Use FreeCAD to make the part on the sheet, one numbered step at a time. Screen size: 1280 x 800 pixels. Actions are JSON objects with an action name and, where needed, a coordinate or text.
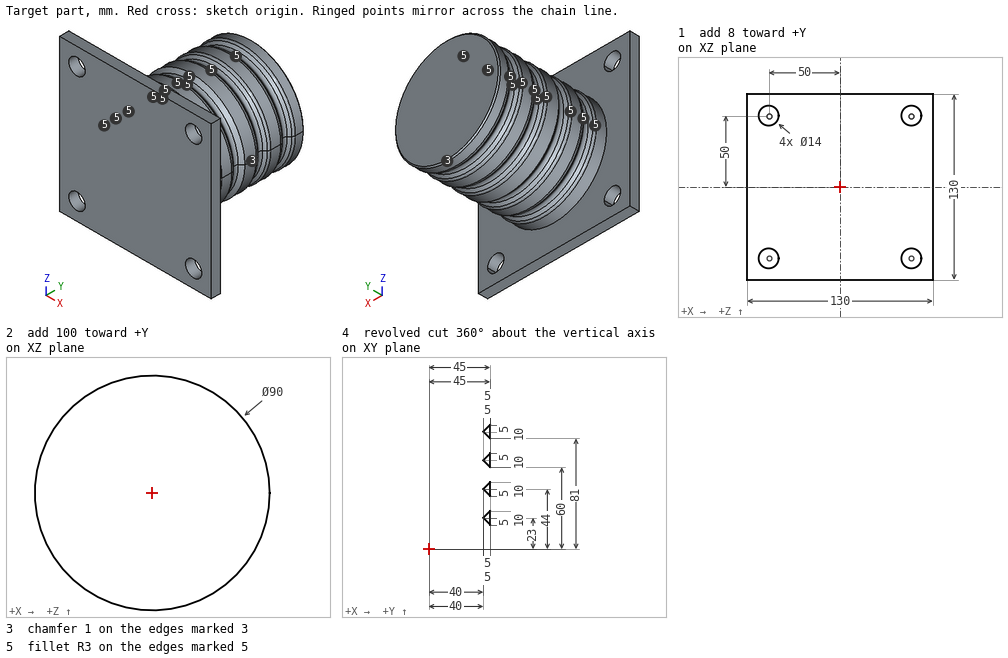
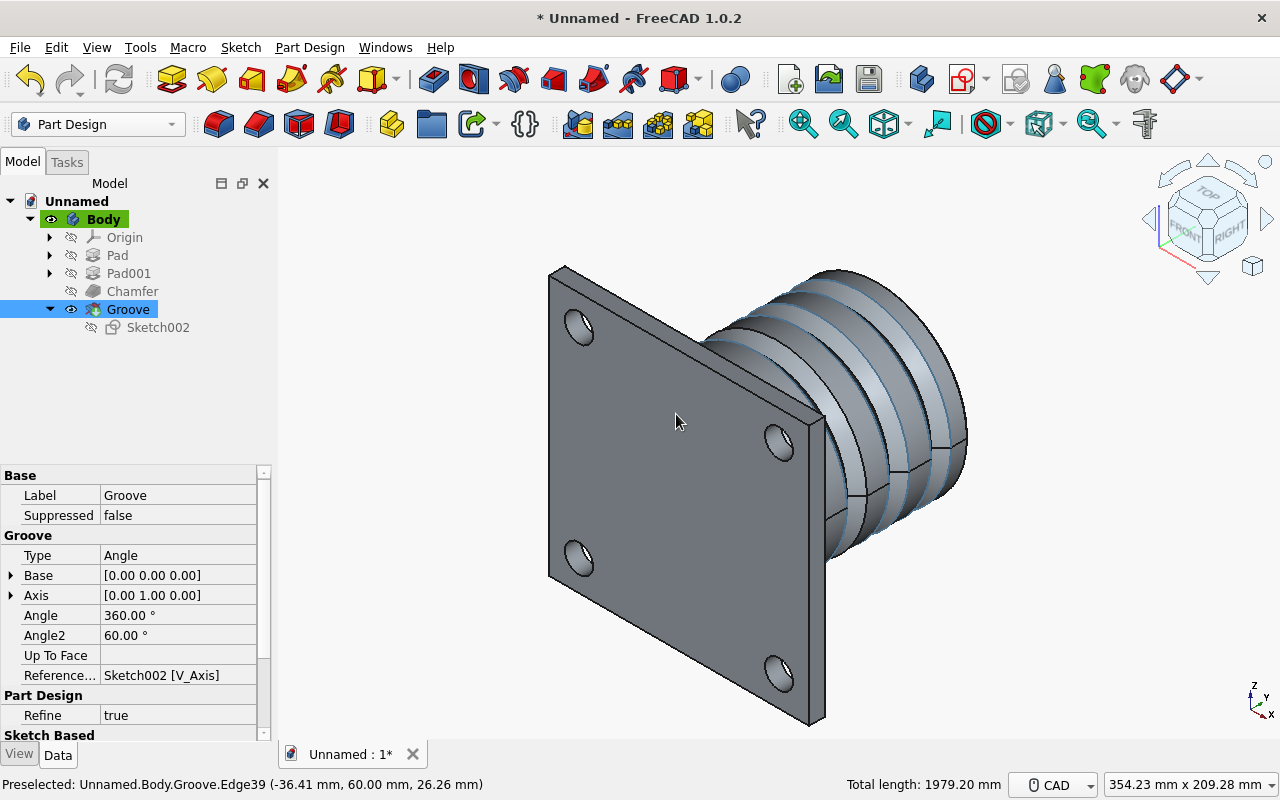
{"action": "key", "text": "1"}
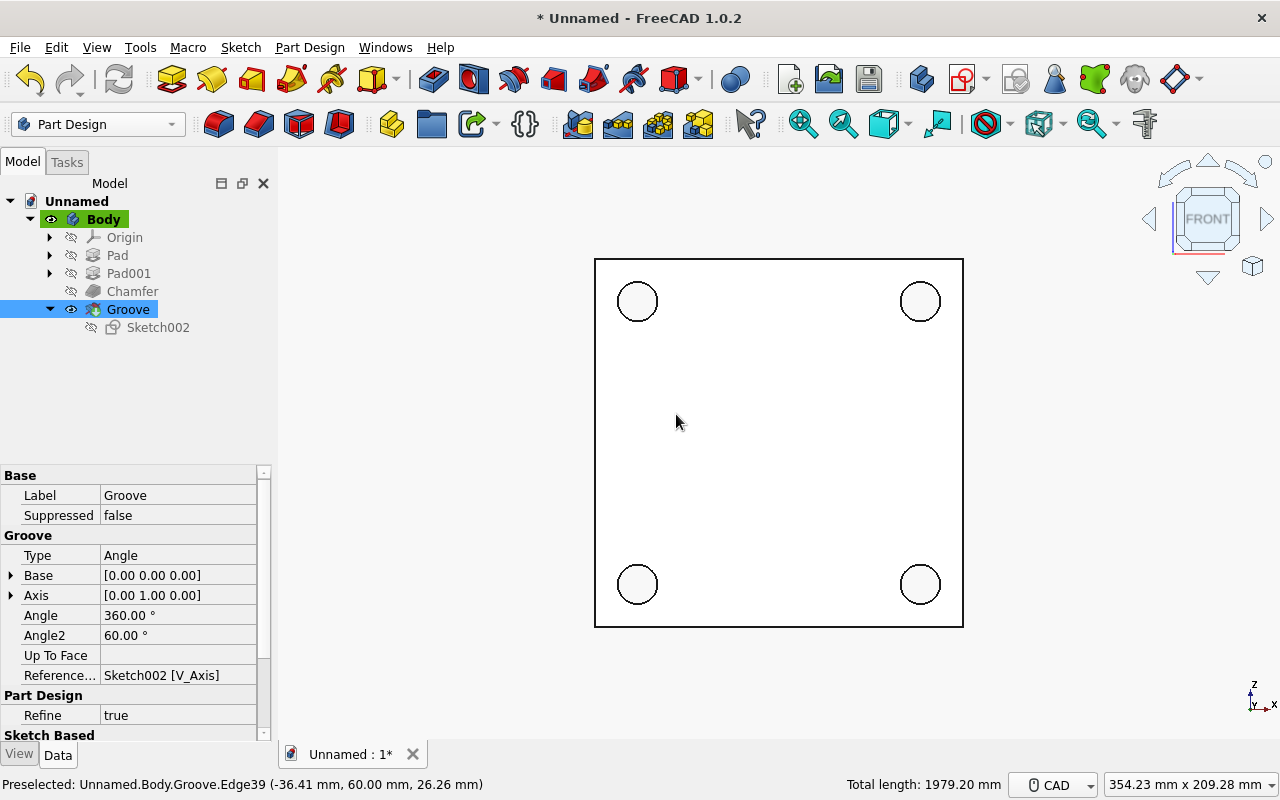
{"action": "key", "text": "3"}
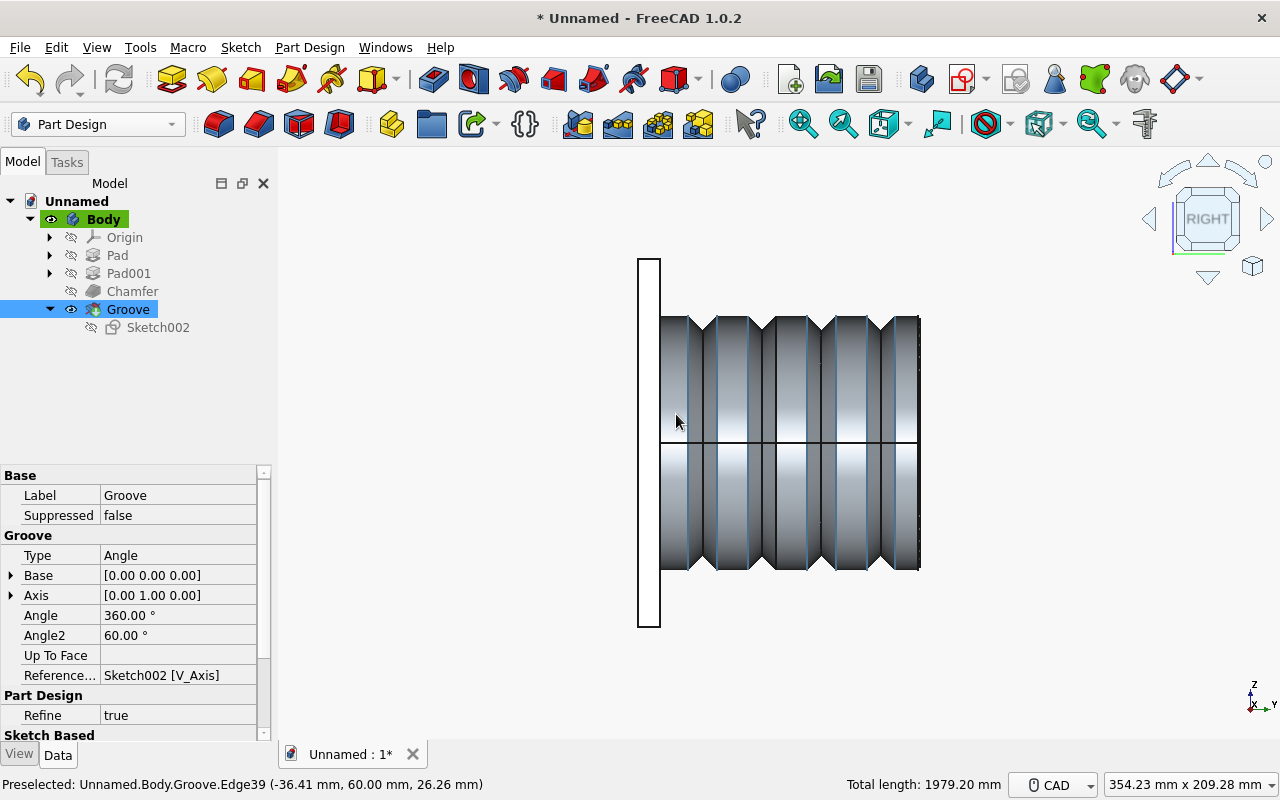
{"action": "key", "text": "5"}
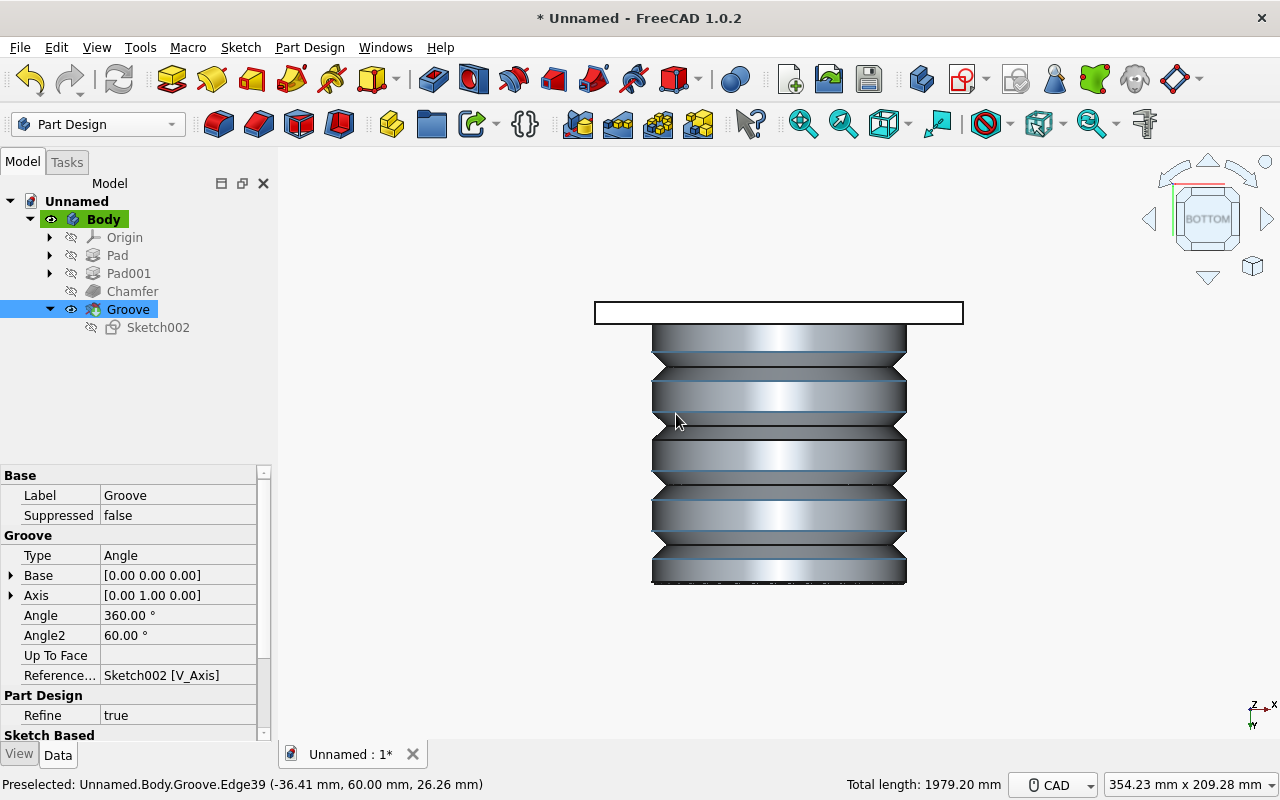
{"action": "key", "text": "4"}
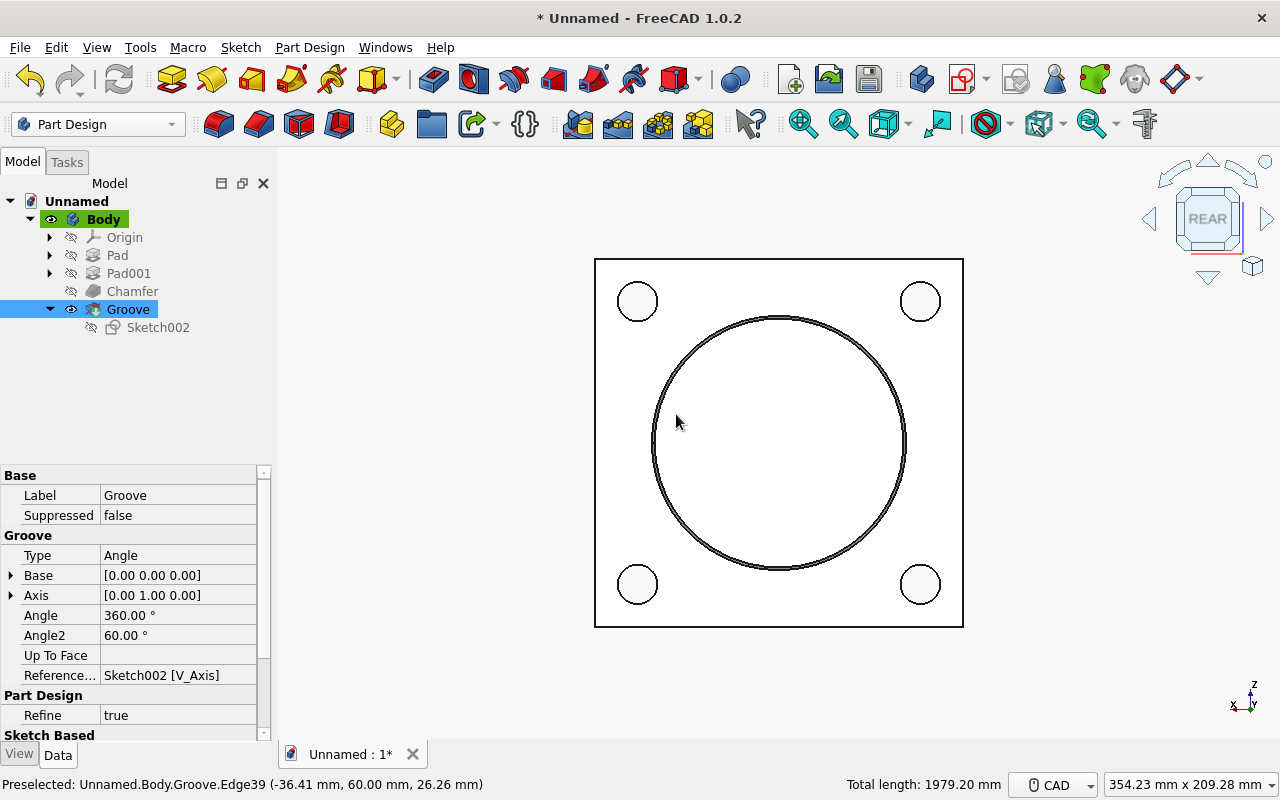
{"action": "key", "text": "6"}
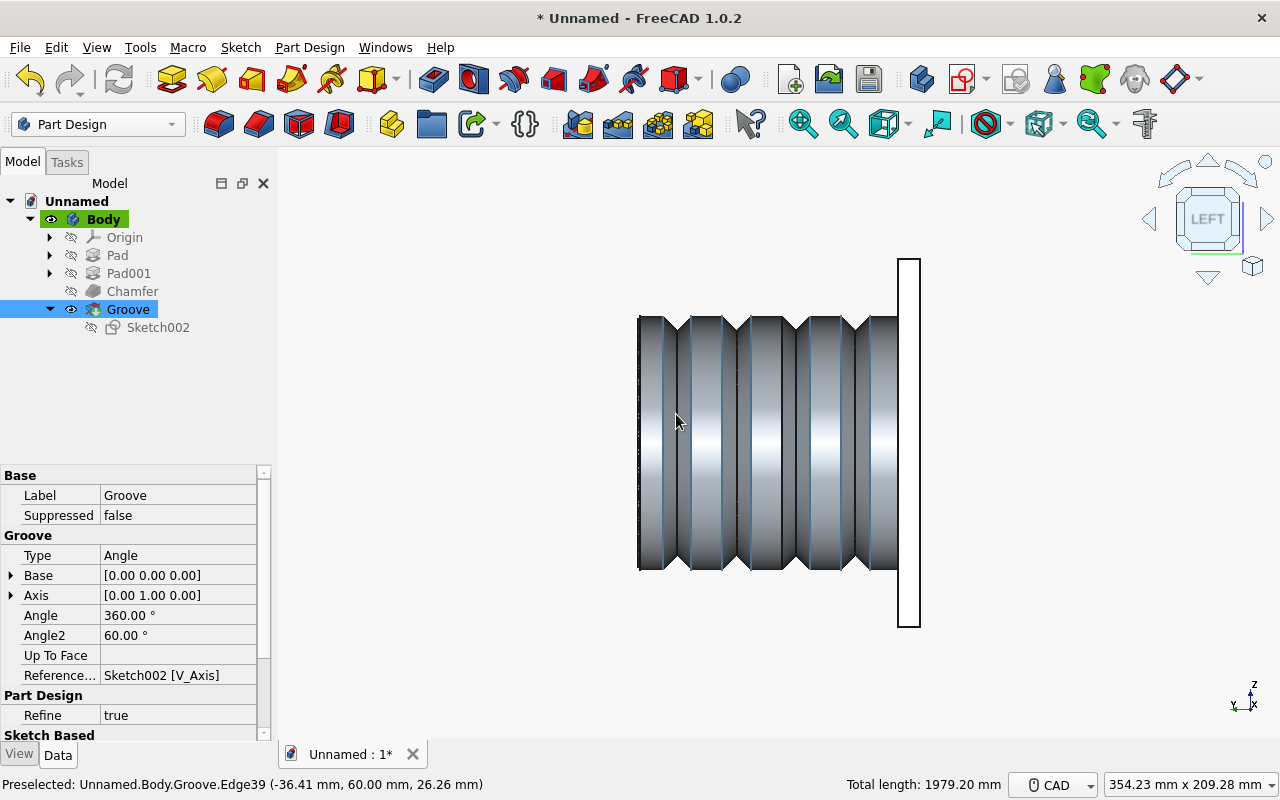
{"action": "key", "text": "v 3"}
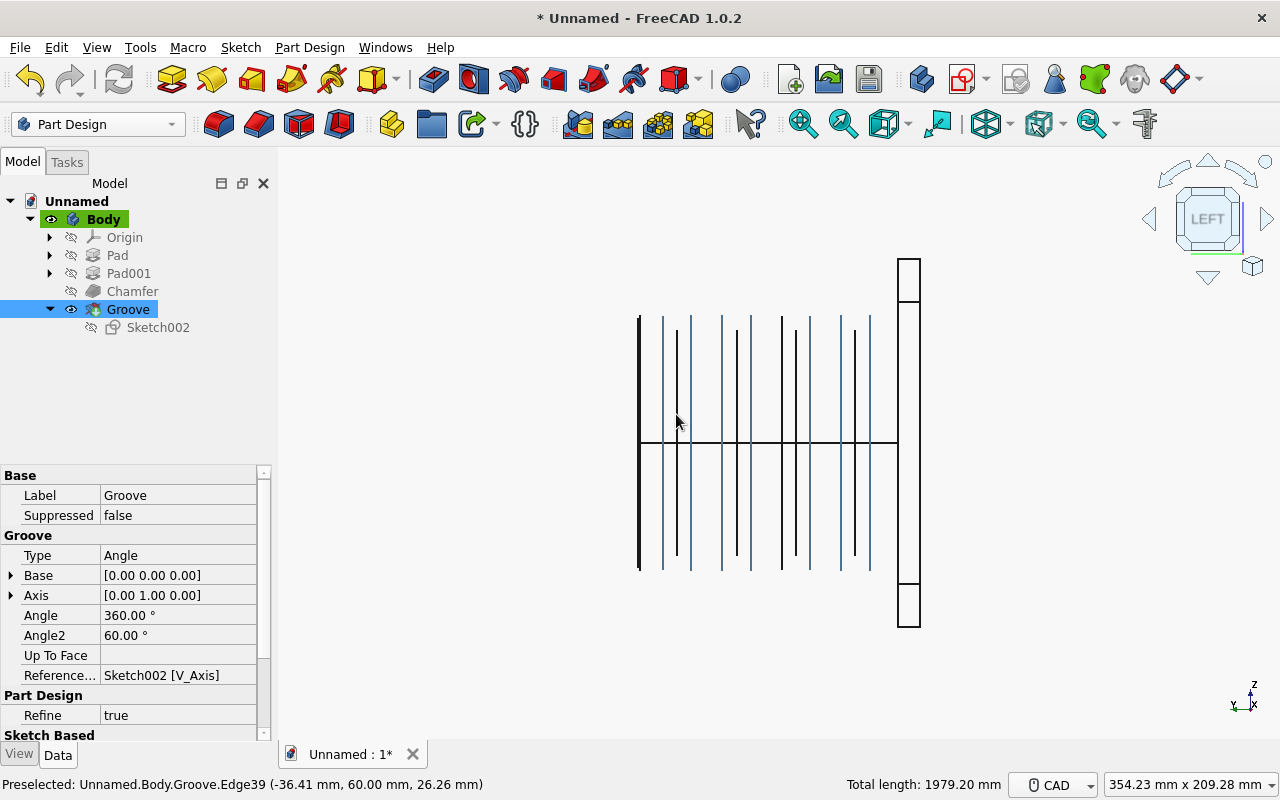
{"action": "key", "text": "0"}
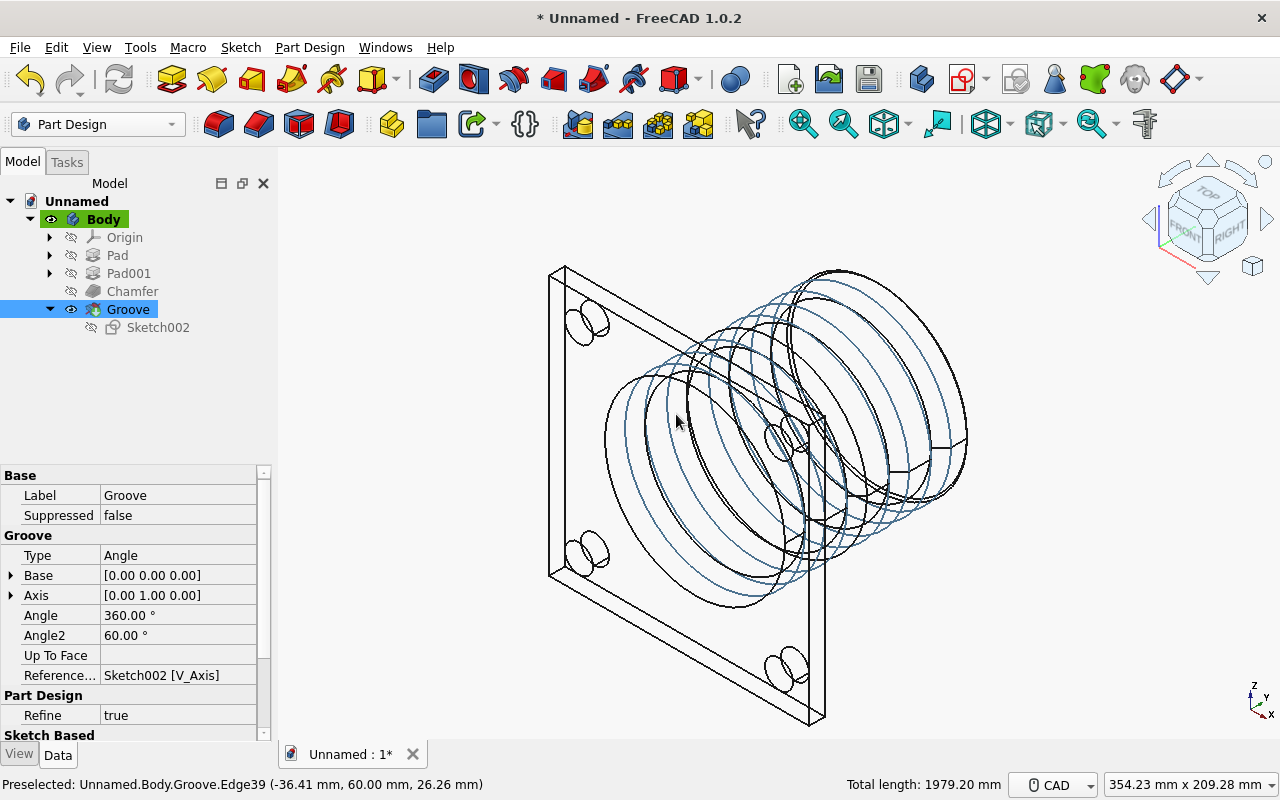
{"action": "left_click", "coordinate": [645, 427], "text": "ctrl"}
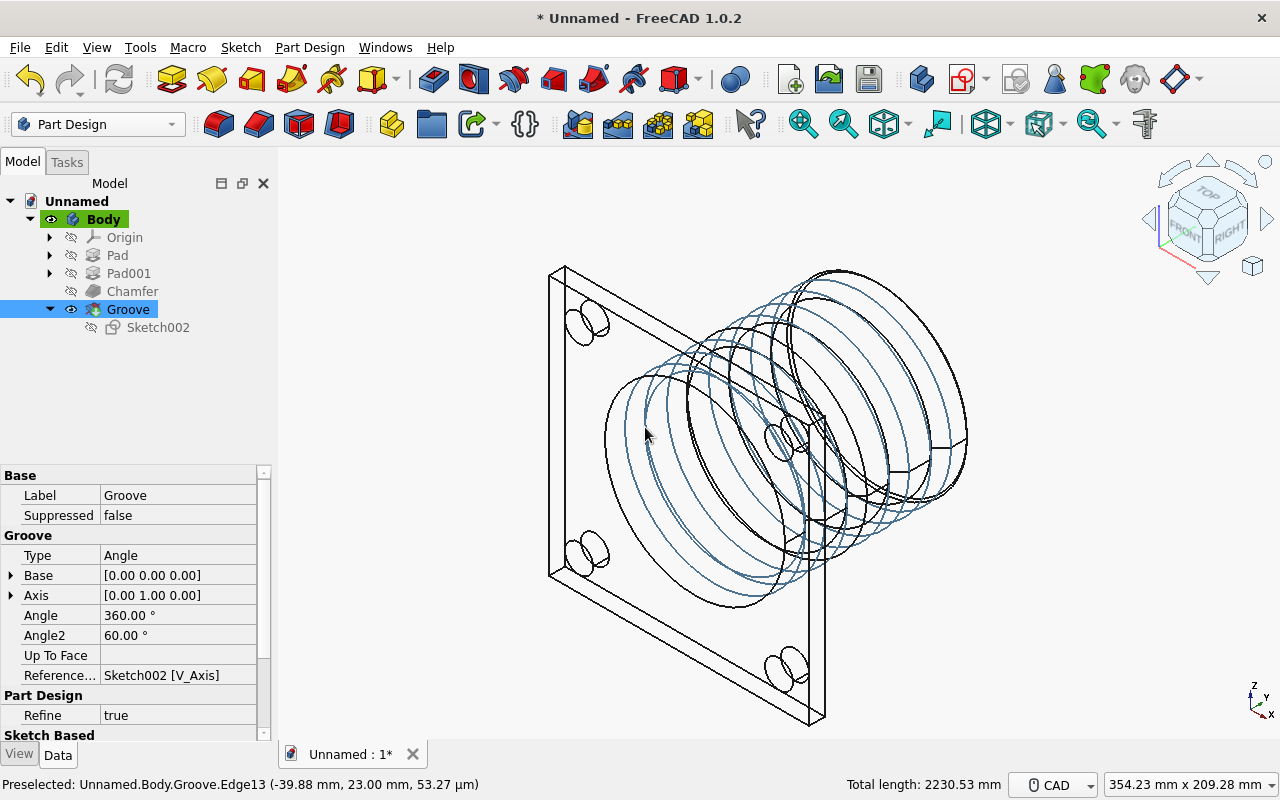
{"action": "left_click", "coordinate": [687, 403], "text": "ctrl"}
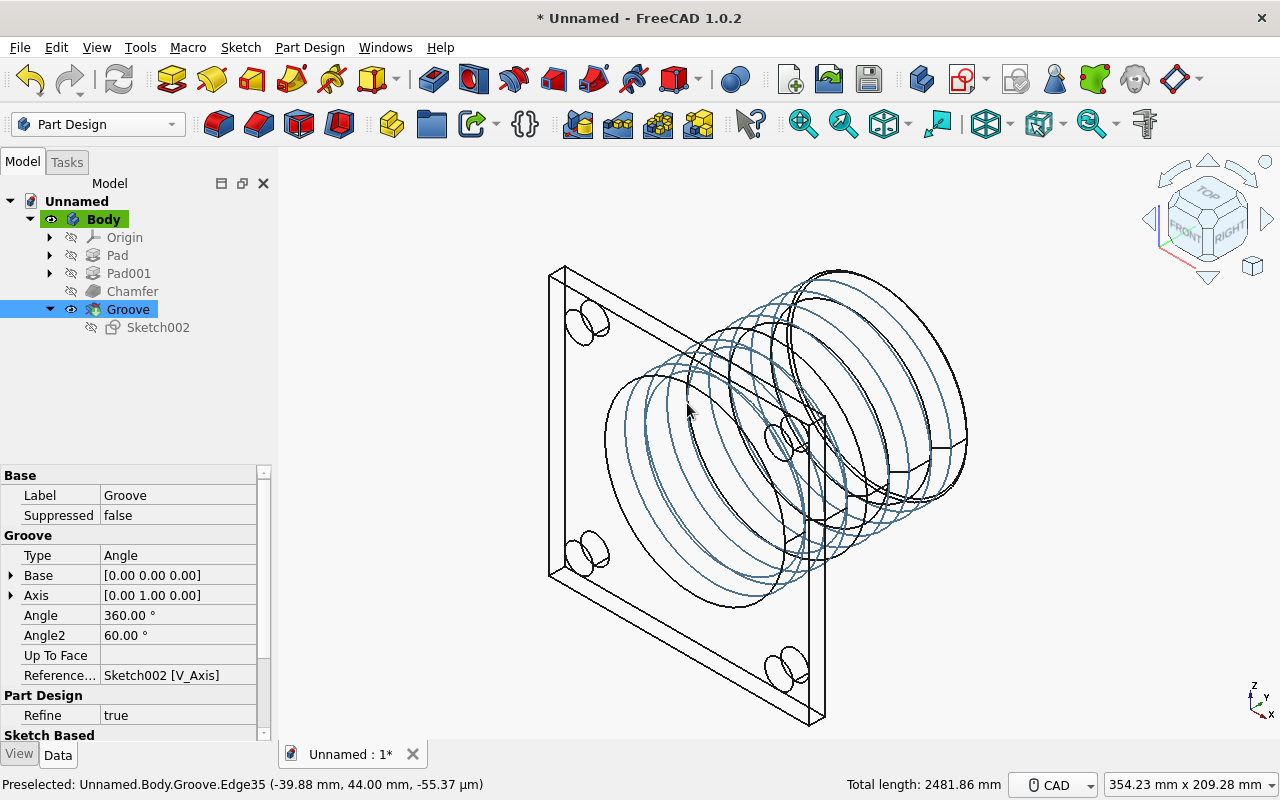
{"action": "scroll", "coordinate": [729, 378], "scroll_direction": "up", "scroll_amount": 6}